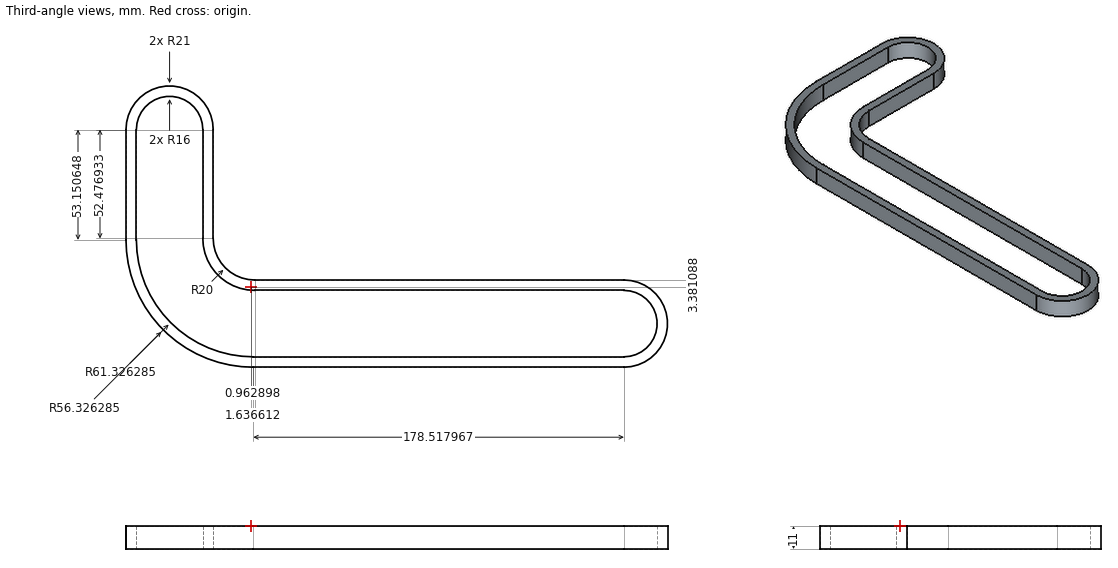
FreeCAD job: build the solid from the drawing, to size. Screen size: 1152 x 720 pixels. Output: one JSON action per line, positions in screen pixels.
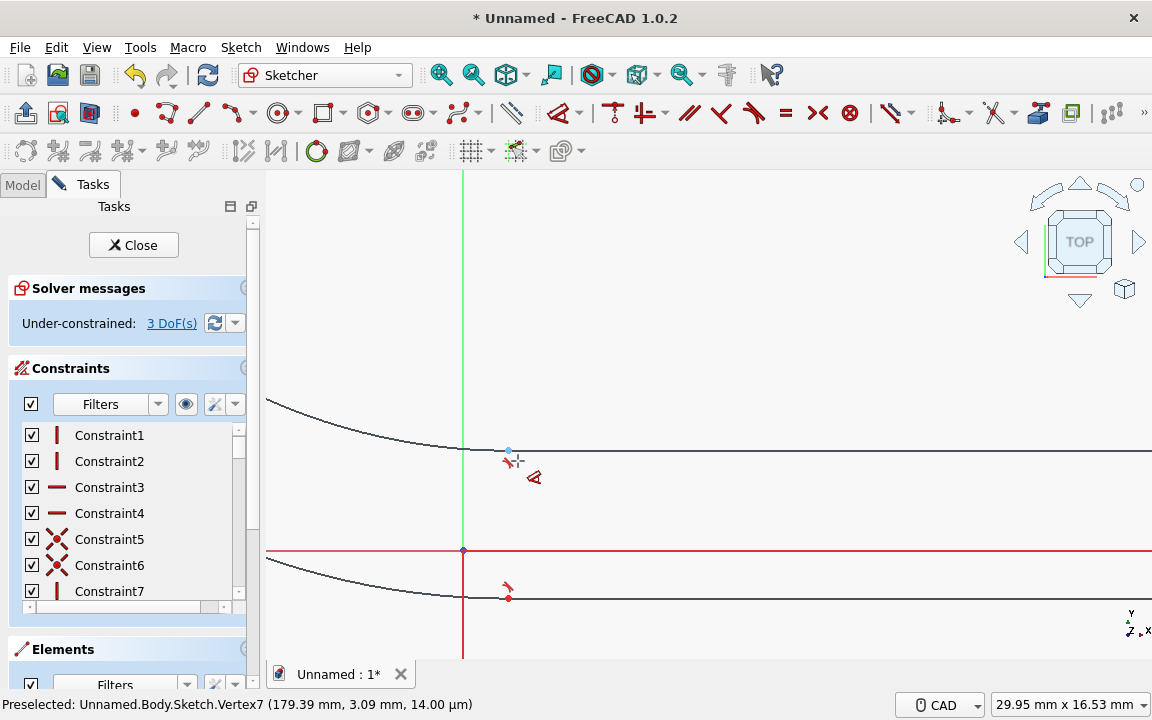
{"action": "left_click", "coordinate": [508, 451]}
{"action": "left_click", "coordinate": [486, 585]}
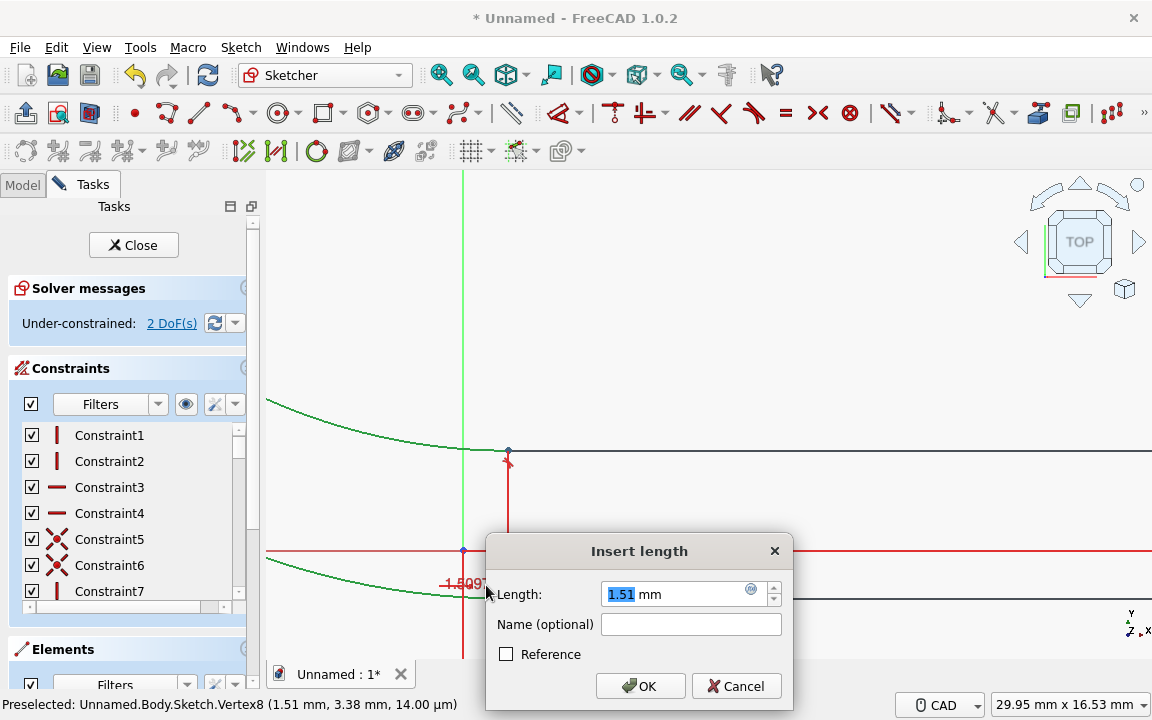
{"action": "type", "text": "1.636612"}
{"action": "key", "text": "Return"}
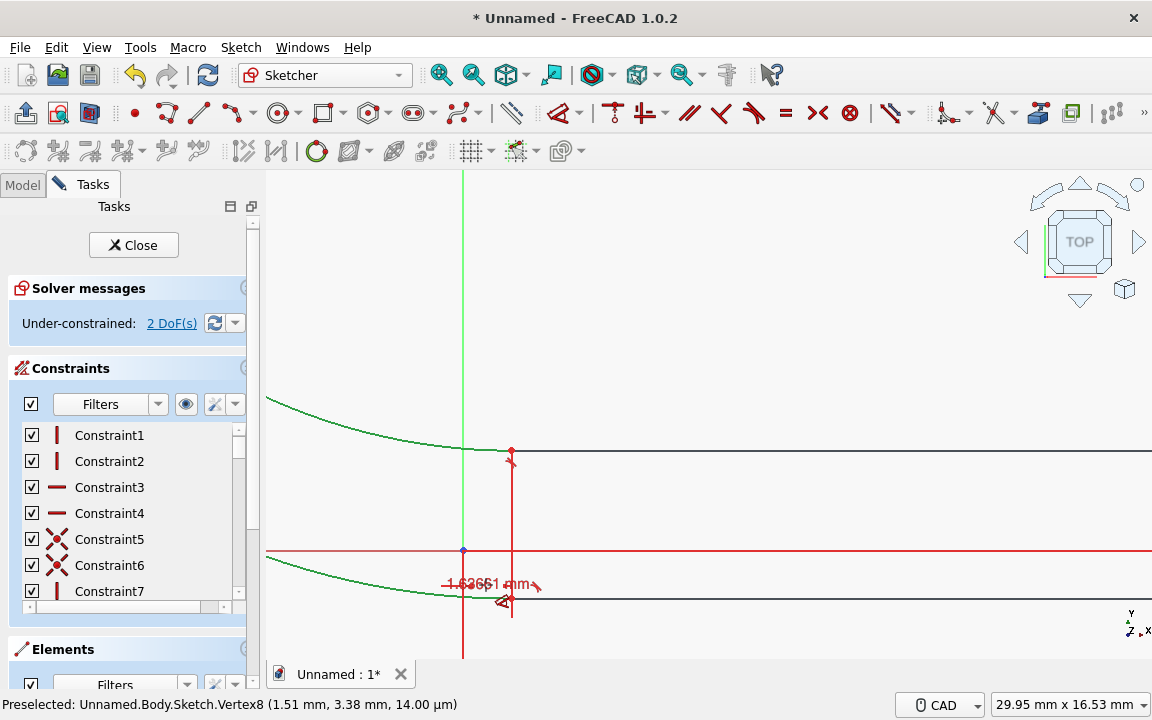
{"action": "scroll", "coordinate": [518, 461], "scroll_direction": "down", "scroll_amount": 14}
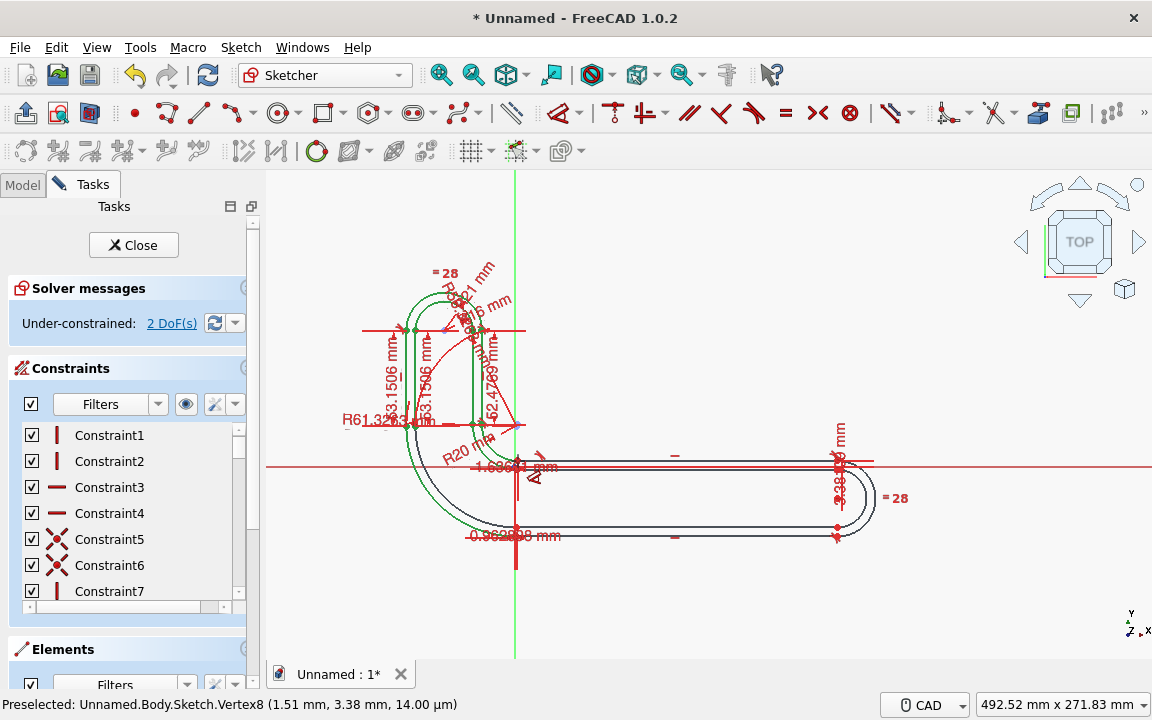
{"action": "scroll", "coordinate": [517, 527], "scroll_direction": "up", "scroll_amount": 16}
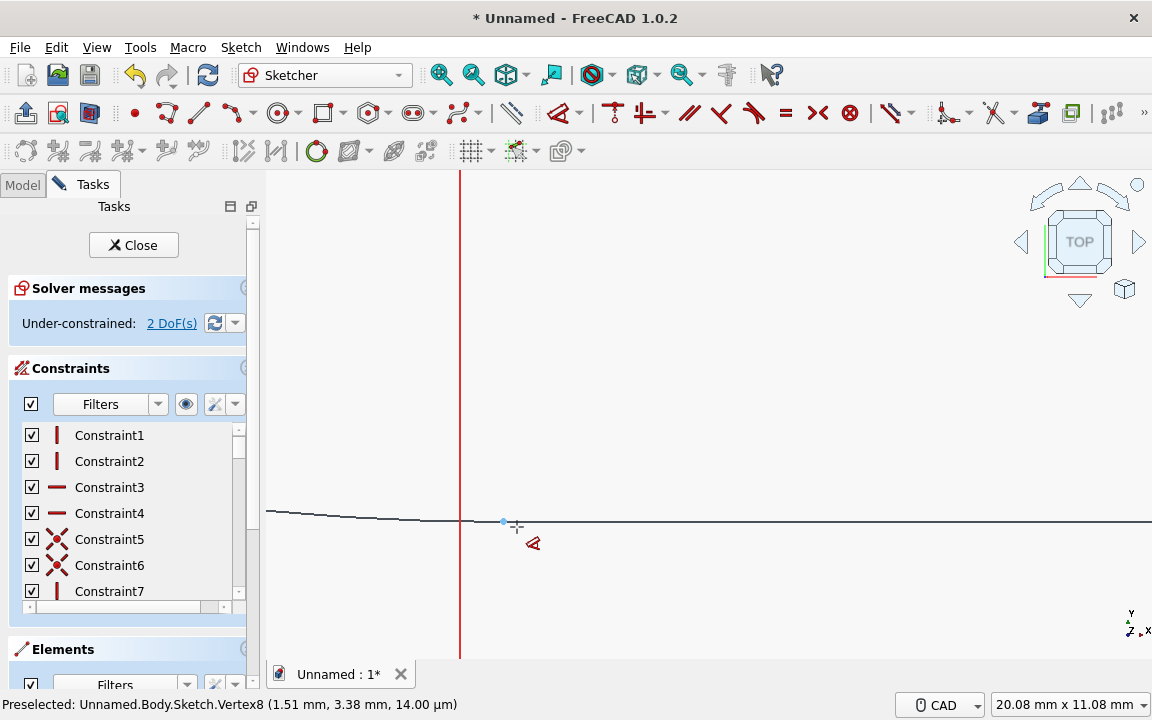
{"action": "left_click", "coordinate": [503, 522]}
{"action": "left_click", "coordinate": [482, 556]}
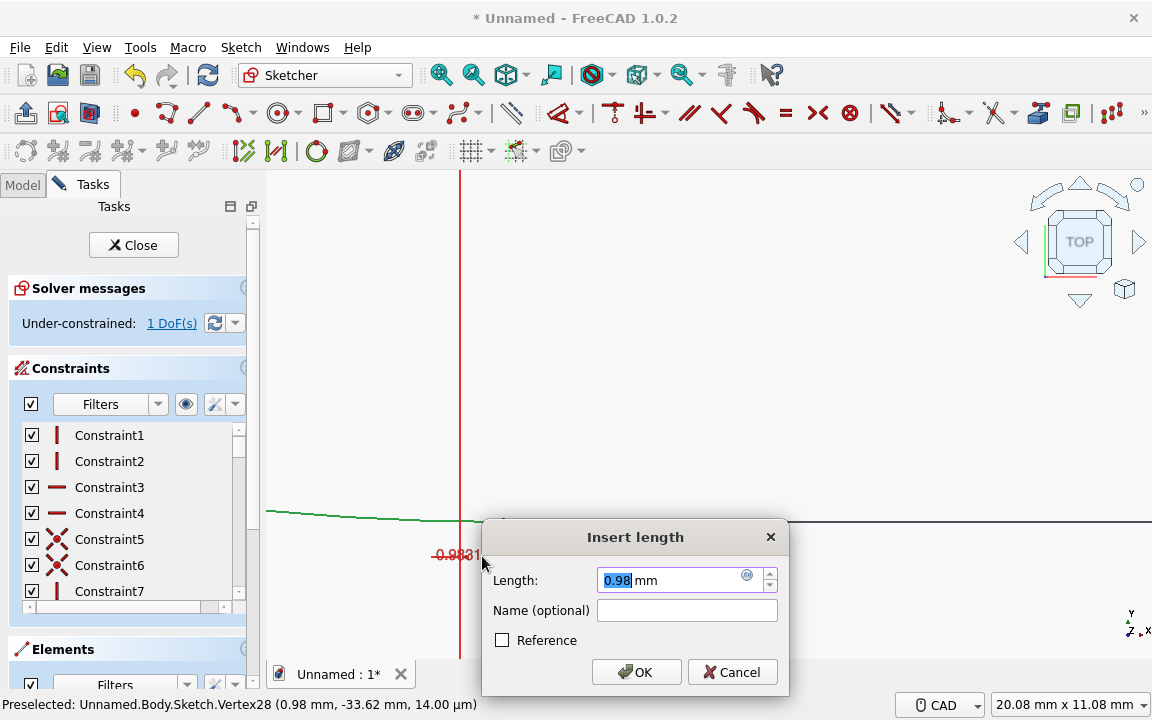
{"action": "type", "text": "0.962898"}
{"action": "key", "text": "Return"}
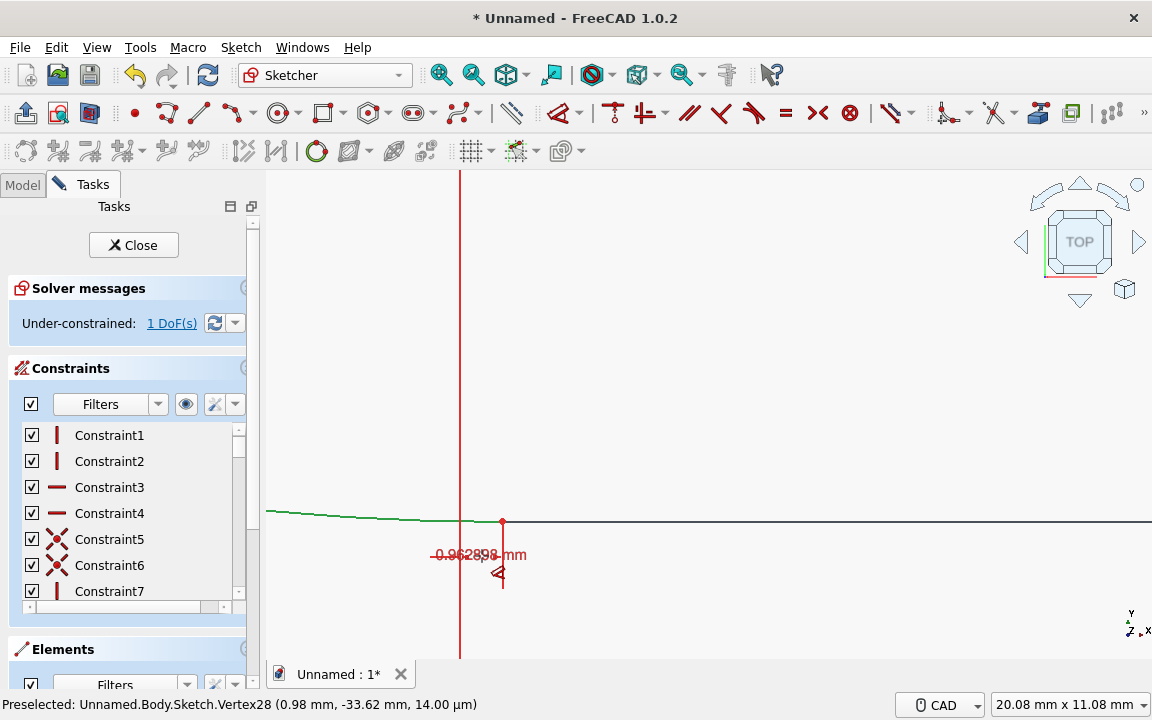
{"action": "scroll", "coordinate": [488, 554], "scroll_direction": "down", "scroll_amount": 15}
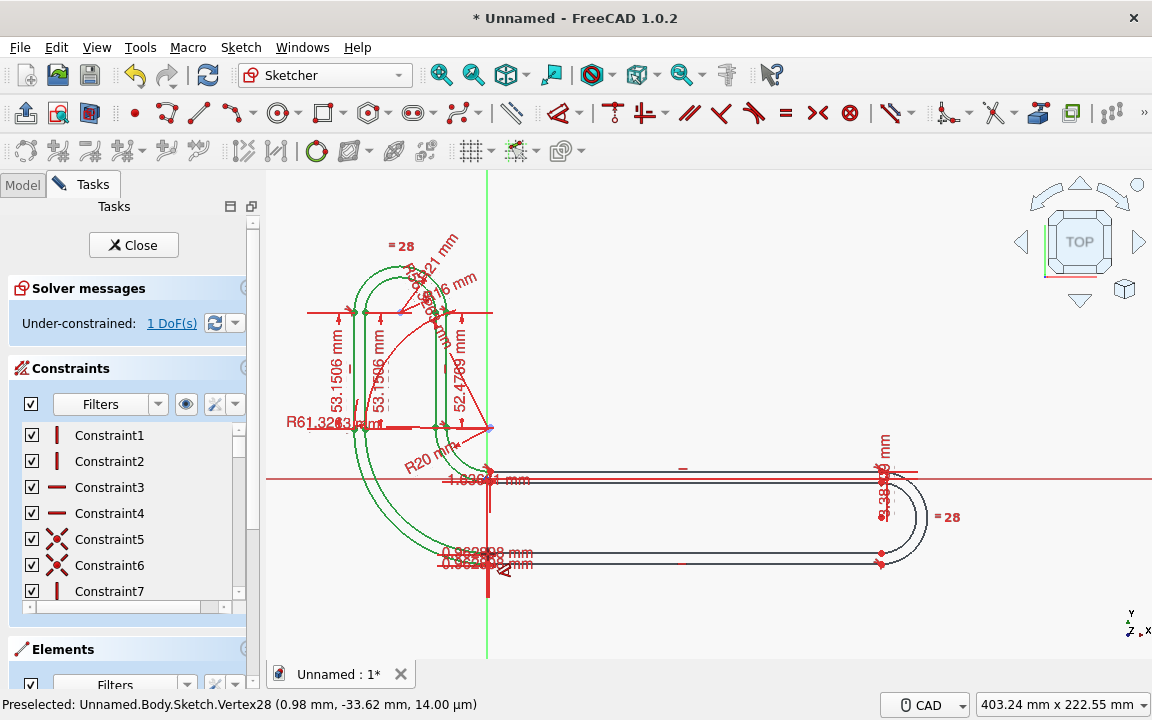
{"action": "scroll", "coordinate": [607, 564], "scroll_direction": "up", "scroll_amount": 2}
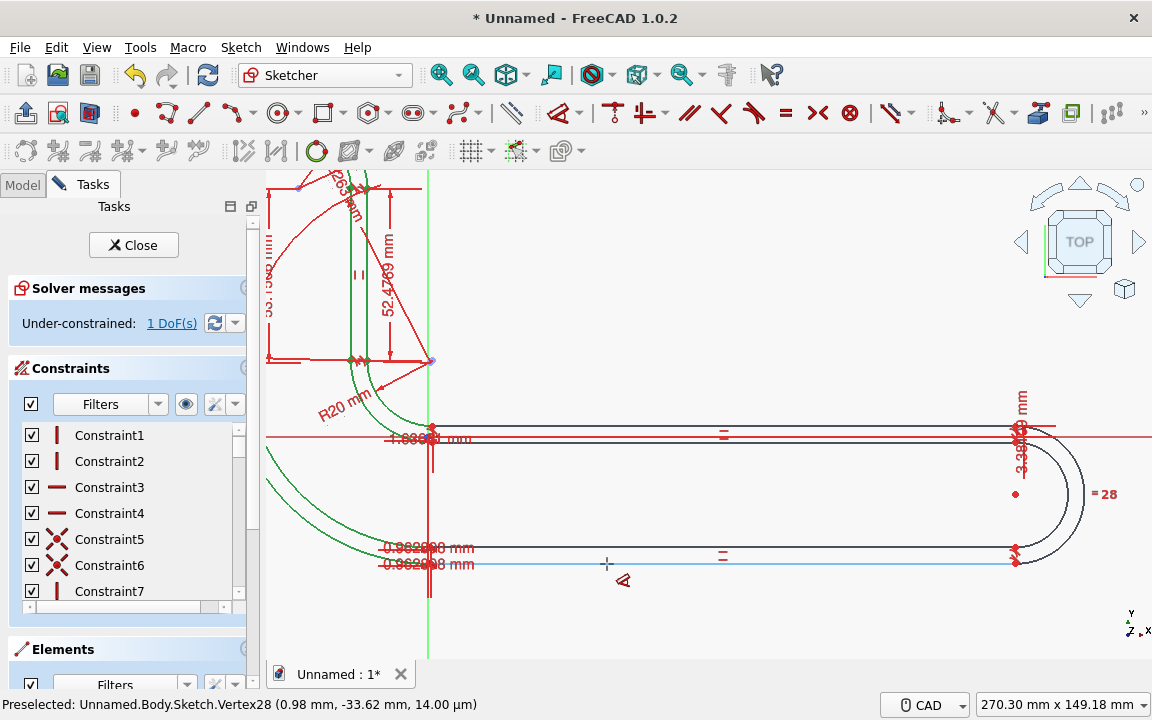
{"action": "left_click", "coordinate": [606, 564]}
{"action": "left_click", "coordinate": [709, 598]}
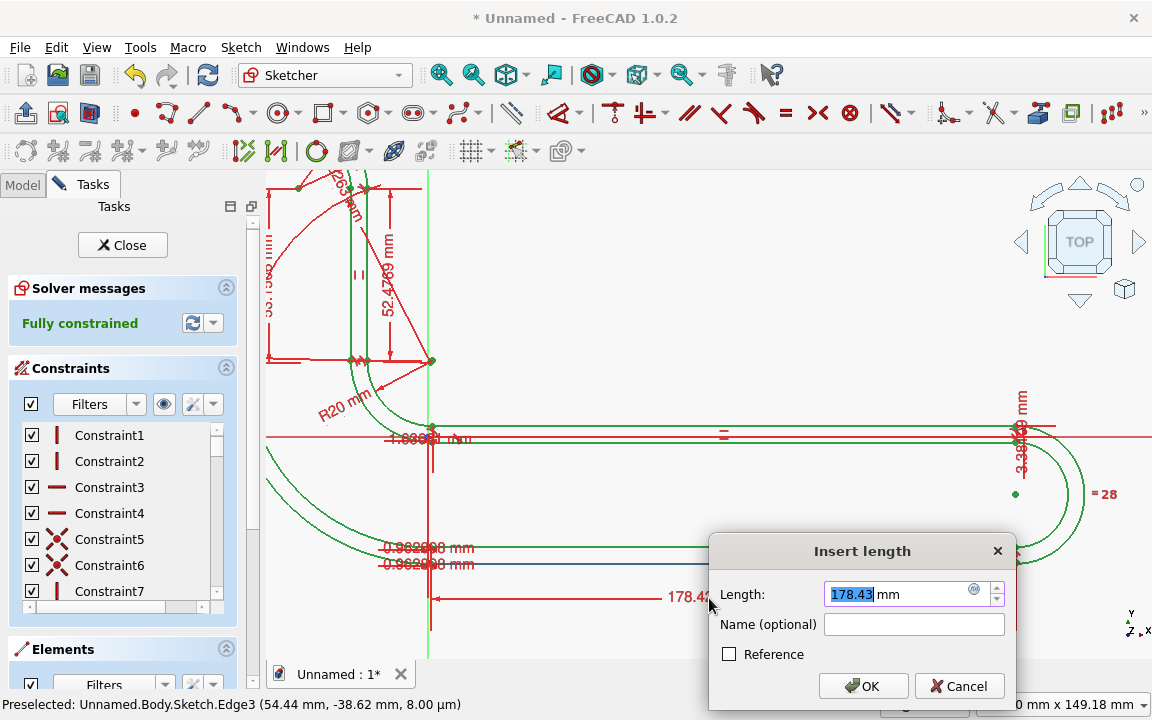
{"action": "type", "text": "178.517967"}
{"action": "key", "text": "Return"}
{"action": "key", "text": "Escape"}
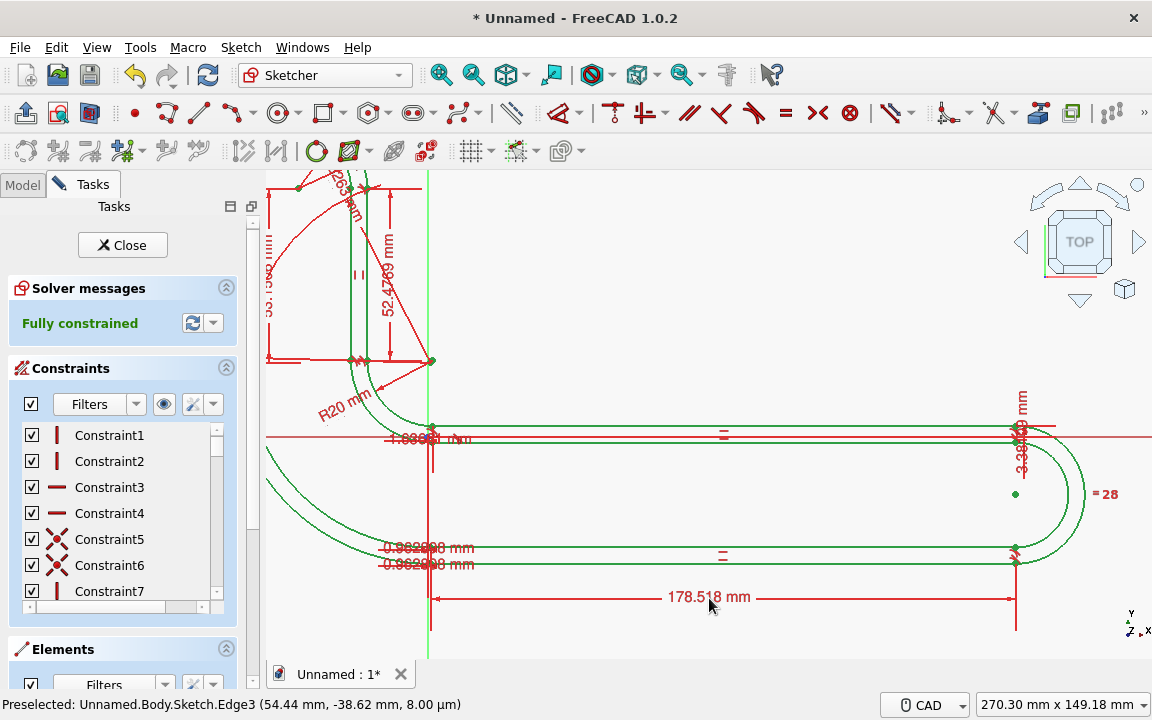
{"action": "left_click", "coordinate": [123, 245]}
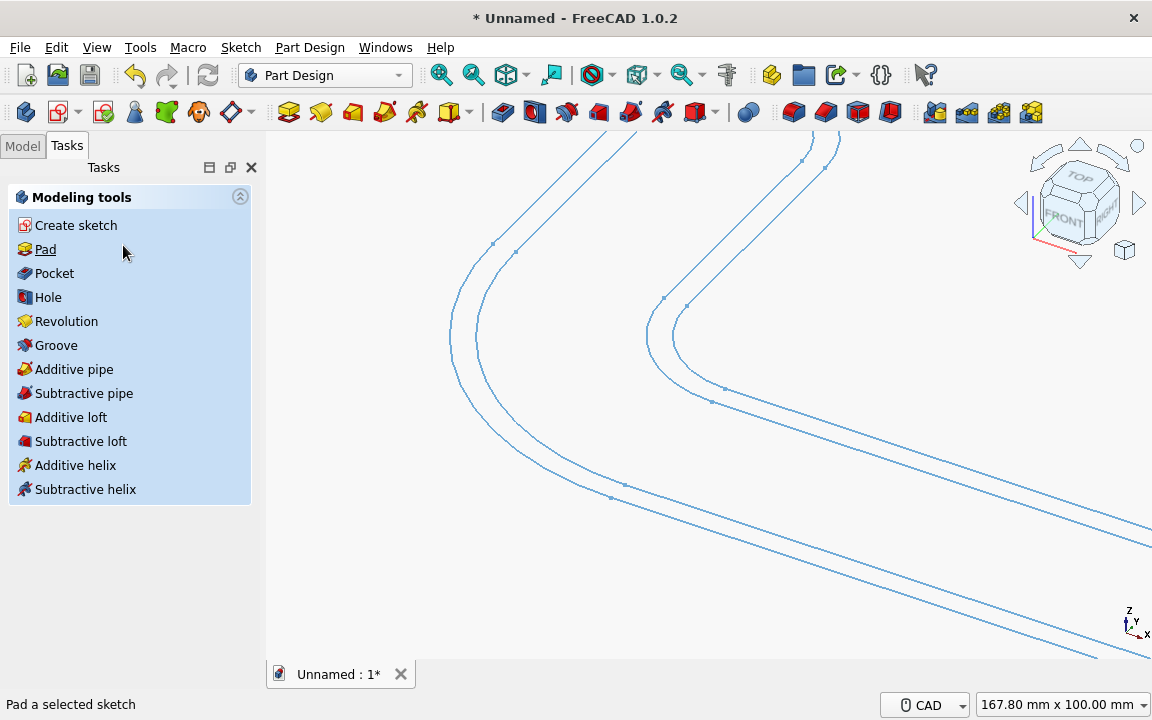
{"action": "left_click", "coordinate": [290, 112]}